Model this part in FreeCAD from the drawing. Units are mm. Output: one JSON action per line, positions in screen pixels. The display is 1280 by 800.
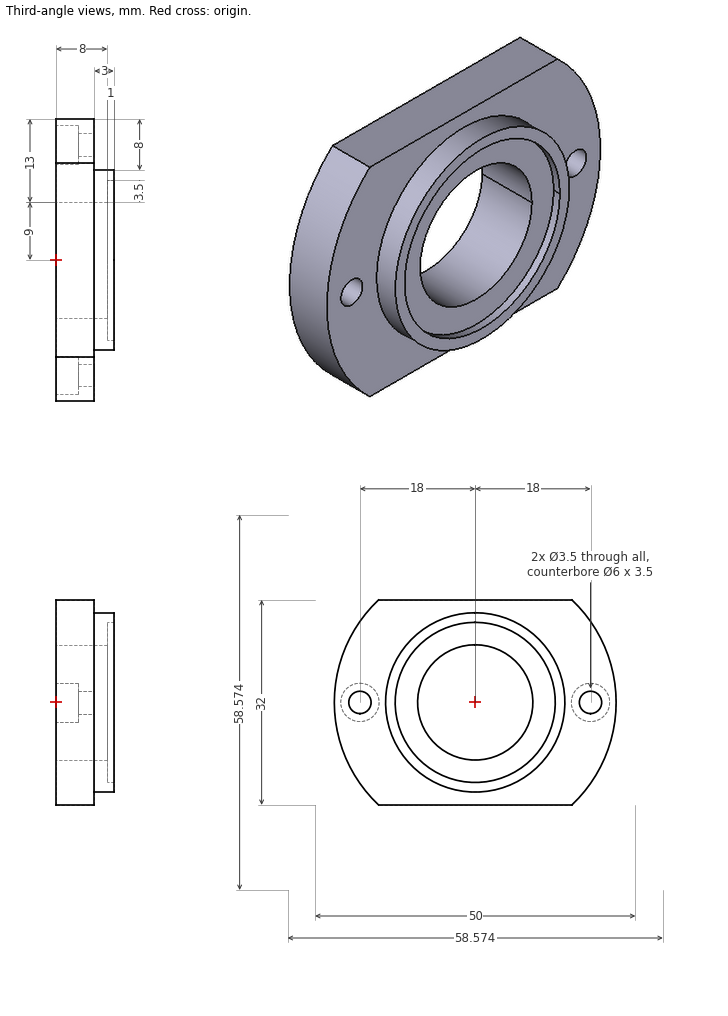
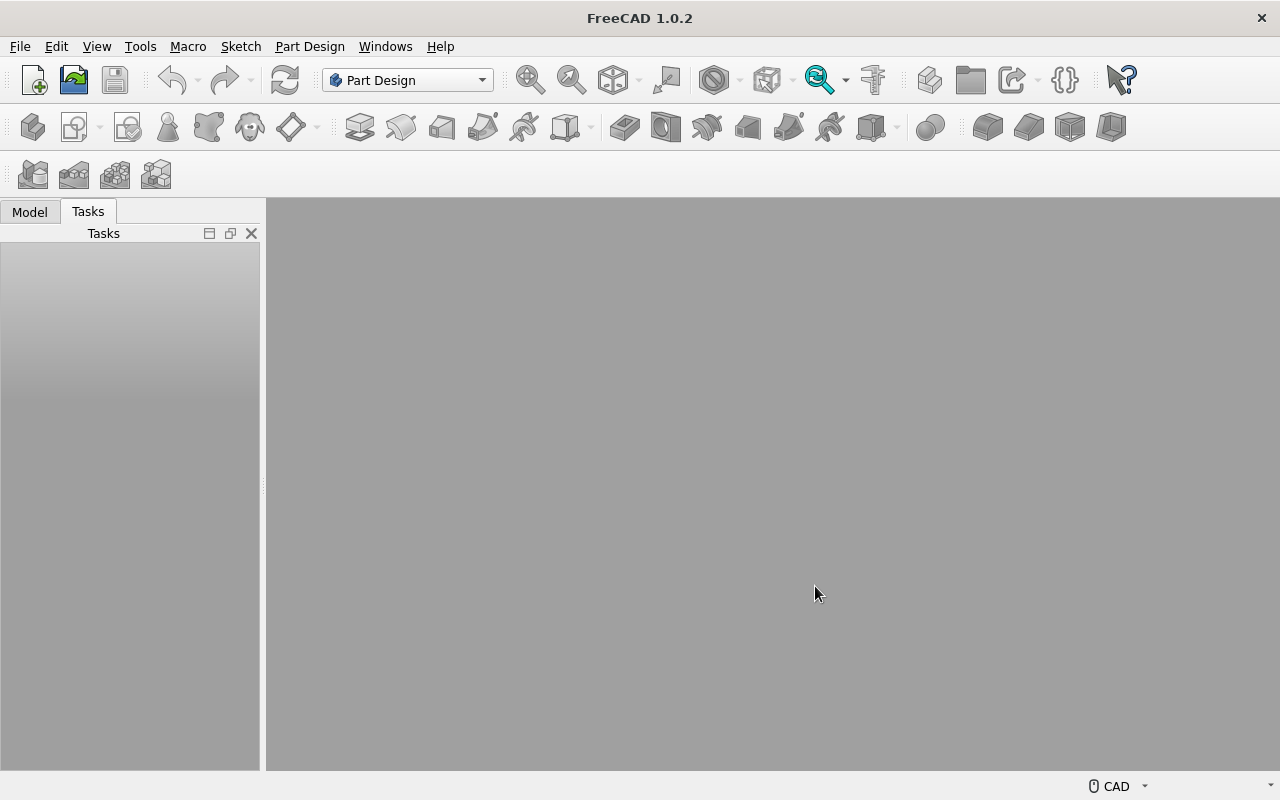
{"action": "left_click", "coordinate": [33, 80]}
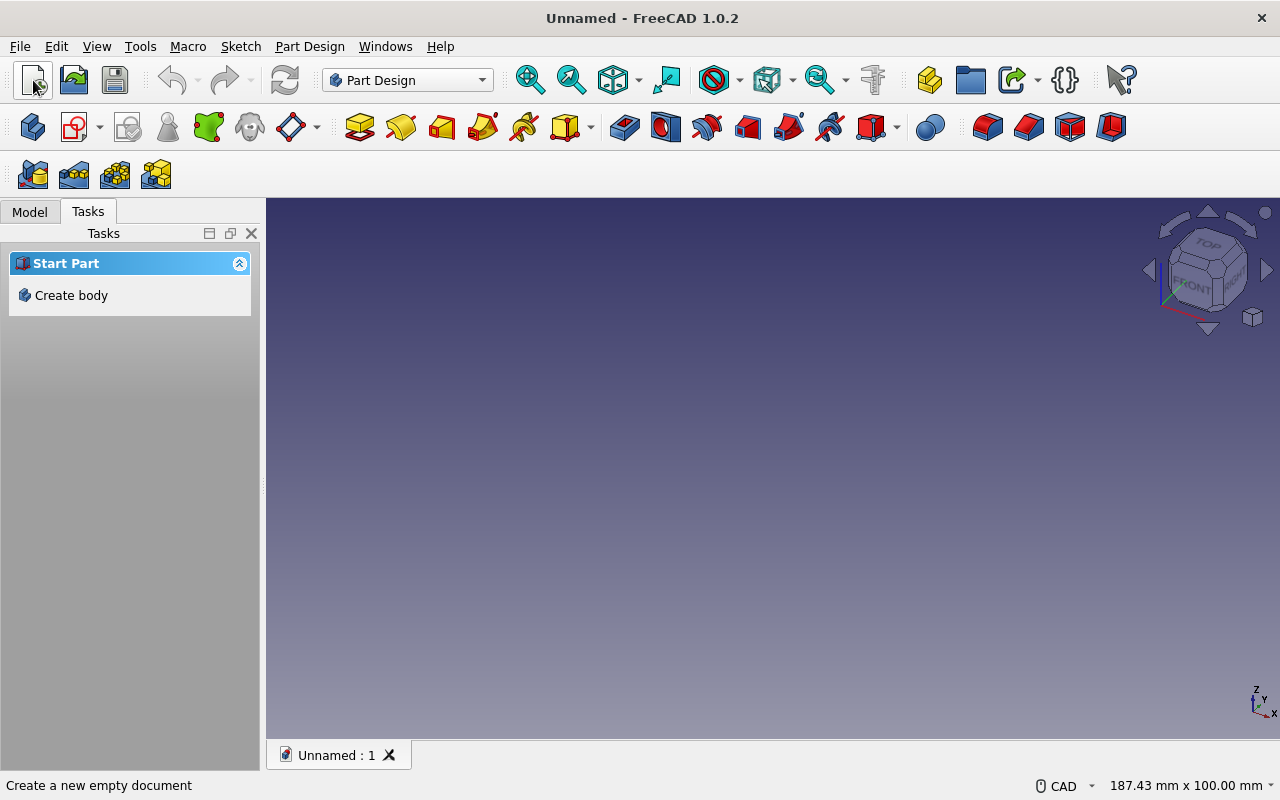
{"action": "left_click", "coordinate": [74, 128]}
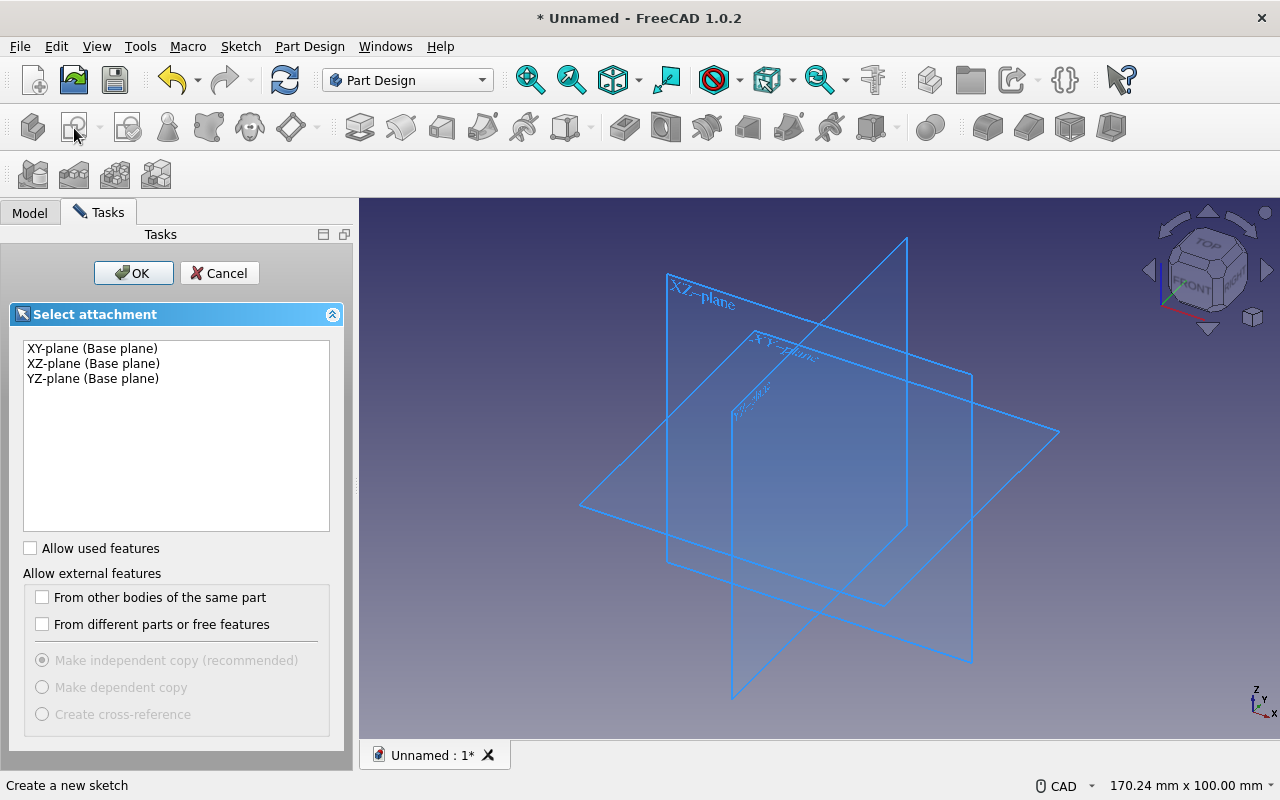
{"action": "left_click", "coordinate": [84, 348]}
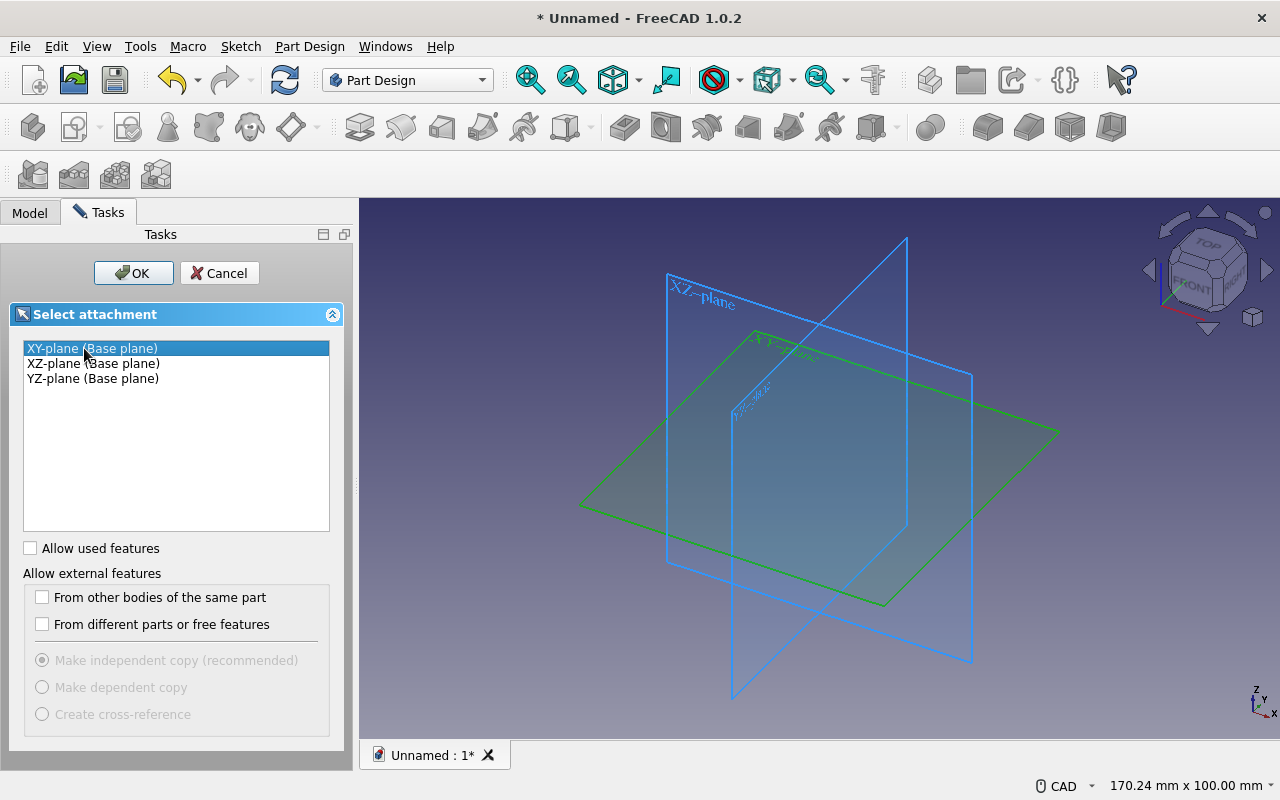
{"action": "left_click", "coordinate": [134, 273]}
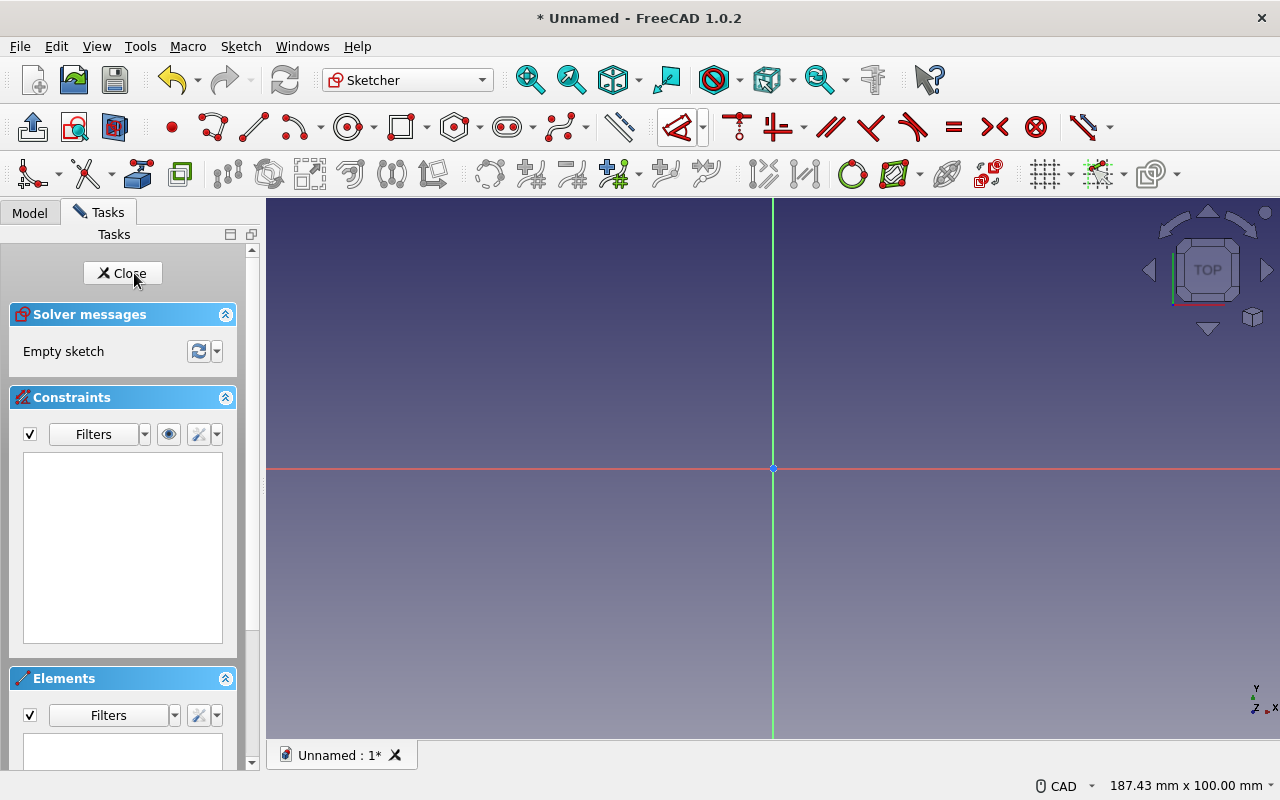
{"action": "scroll", "coordinate": [851, 374], "scroll_direction": "up", "scroll_amount": 5}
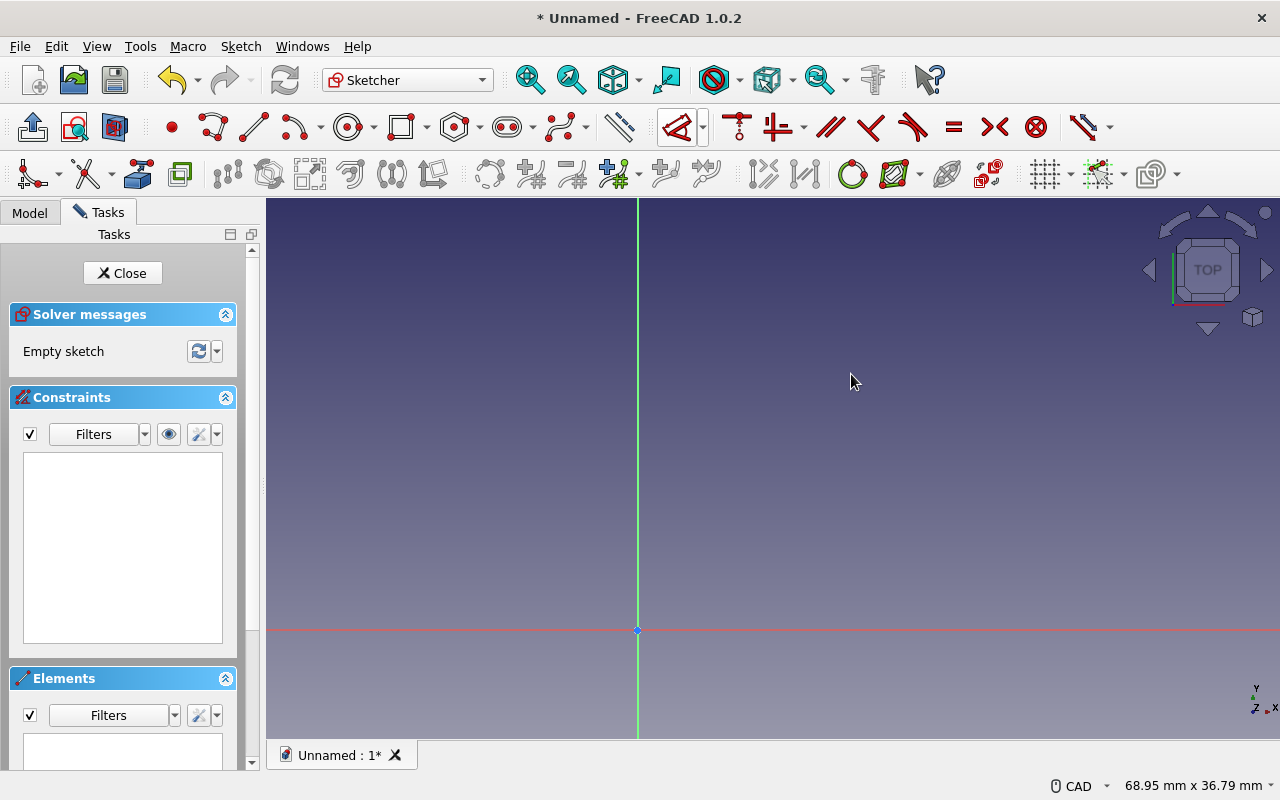
{"action": "left_click", "coordinate": [213, 128]}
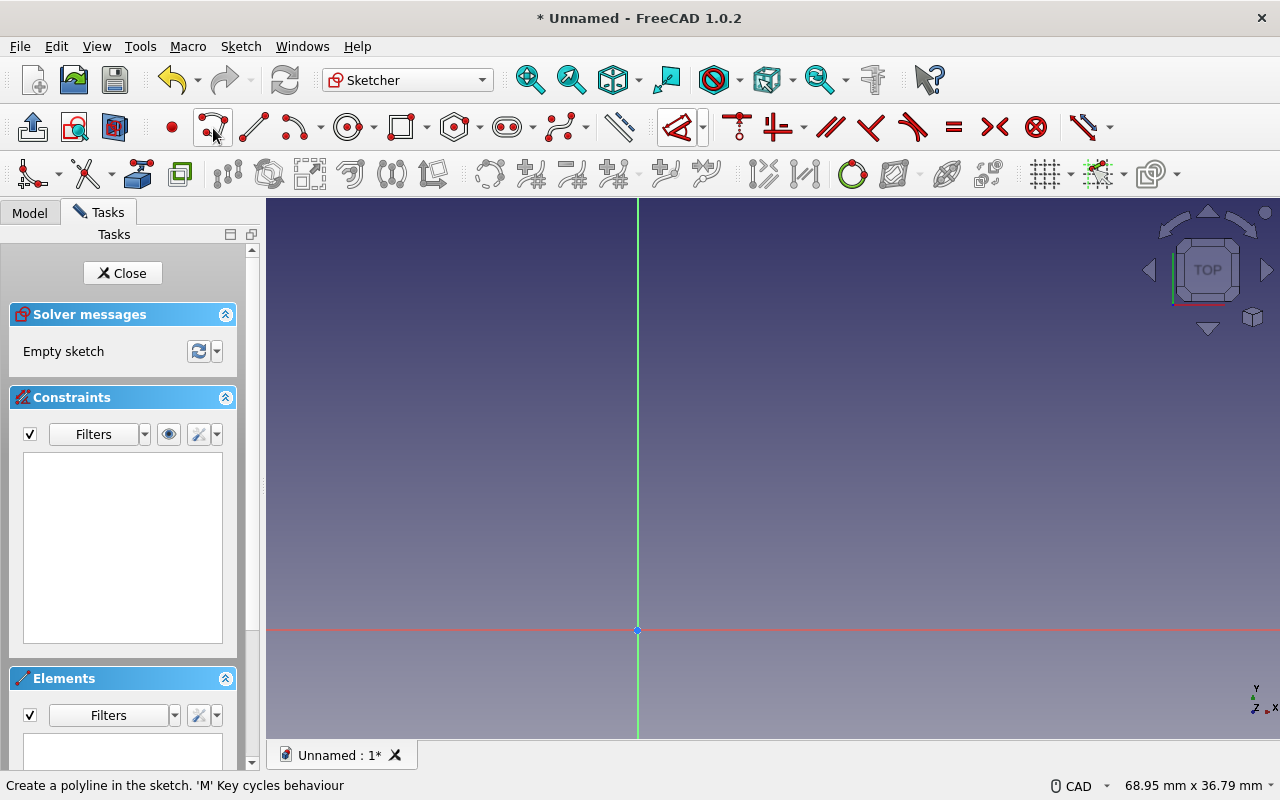
{"action": "left_click", "coordinate": [638, 498]}
{"action": "left_click", "coordinate": [756, 498]}
{"action": "left_click", "coordinate": [756, 446]}
{"action": "left_click", "coordinate": [770, 446]}
{"action": "left_click", "coordinate": [770, 424]}
{"action": "left_click", "coordinate": [726, 424]}
{"action": "left_click", "coordinate": [726, 307]}
{"action": "left_click", "coordinate": [647, 307]}
{"action": "left_click", "coordinate": [638, 499]}
{"action": "key", "text": "Escape"}
{"action": "key", "text": "Escape"}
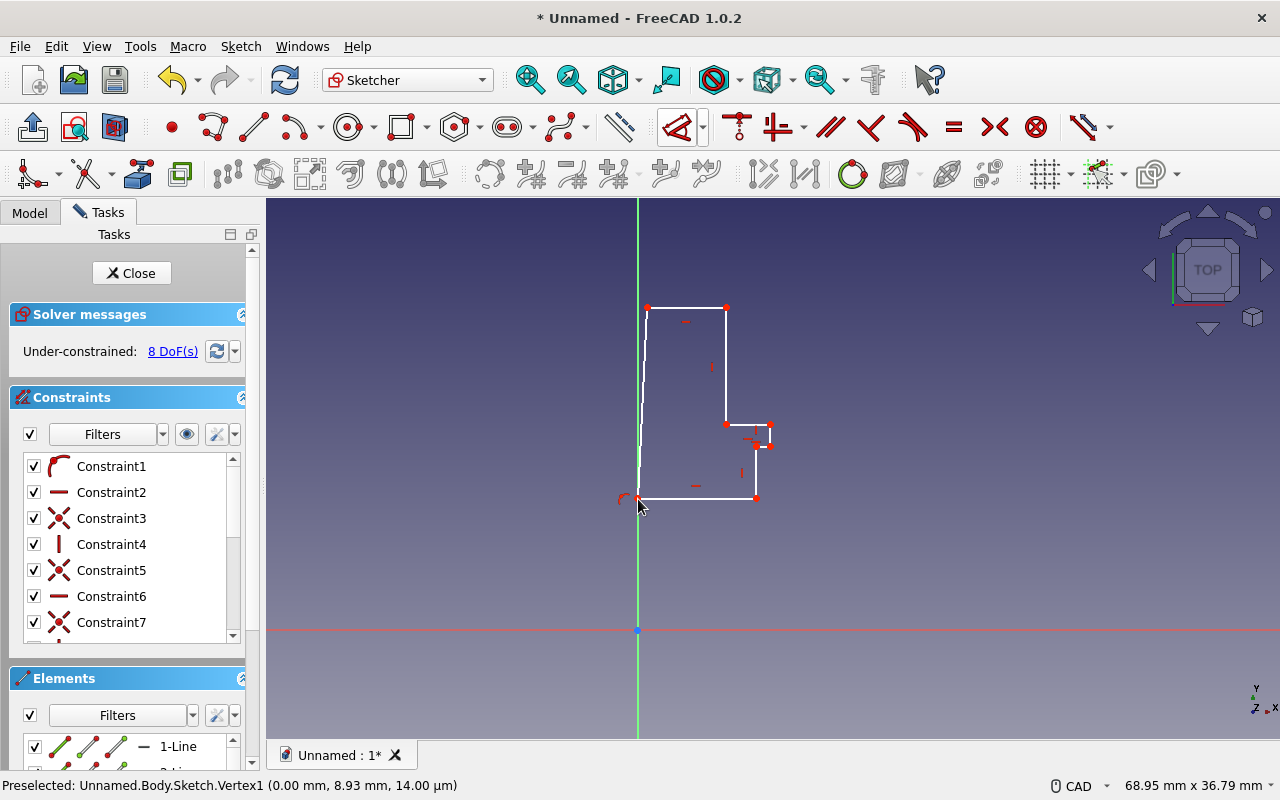
{"action": "left_click", "coordinate": [641, 442]}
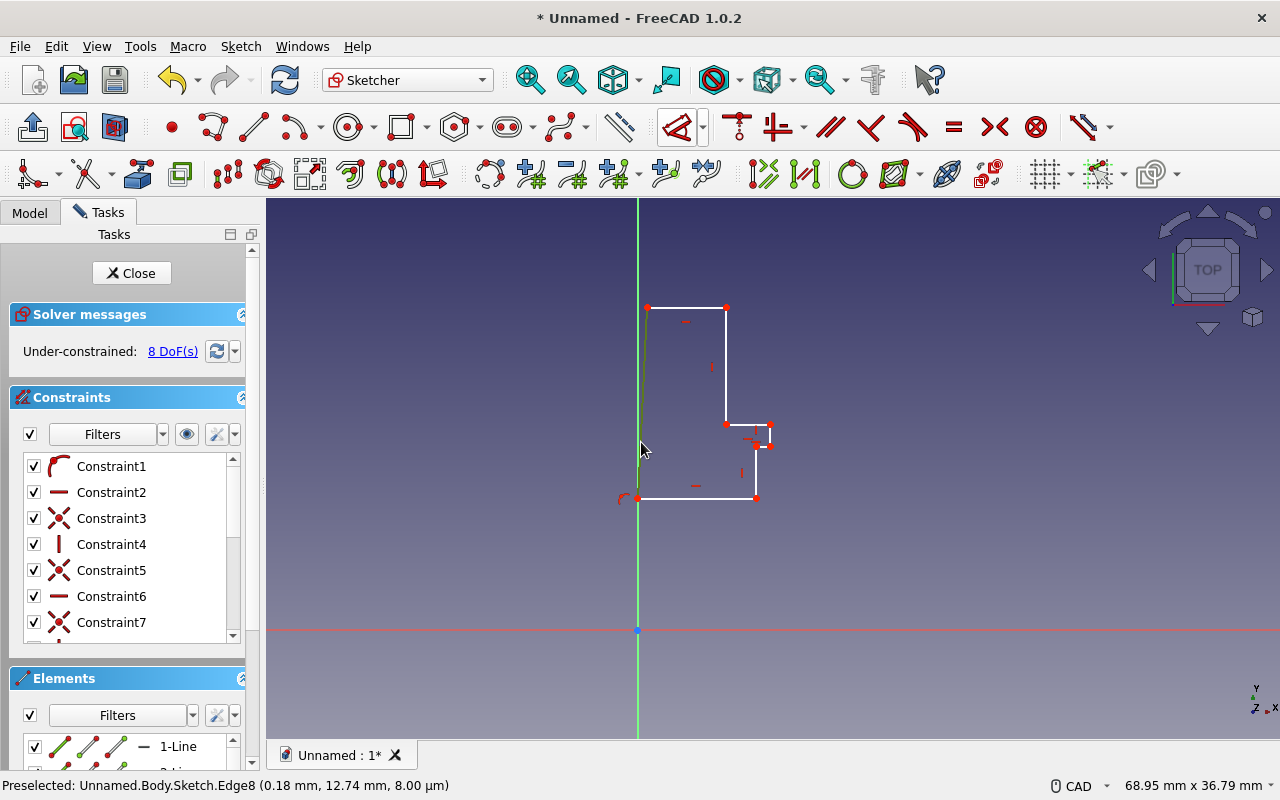
{"action": "left_click", "coordinate": [804, 128]}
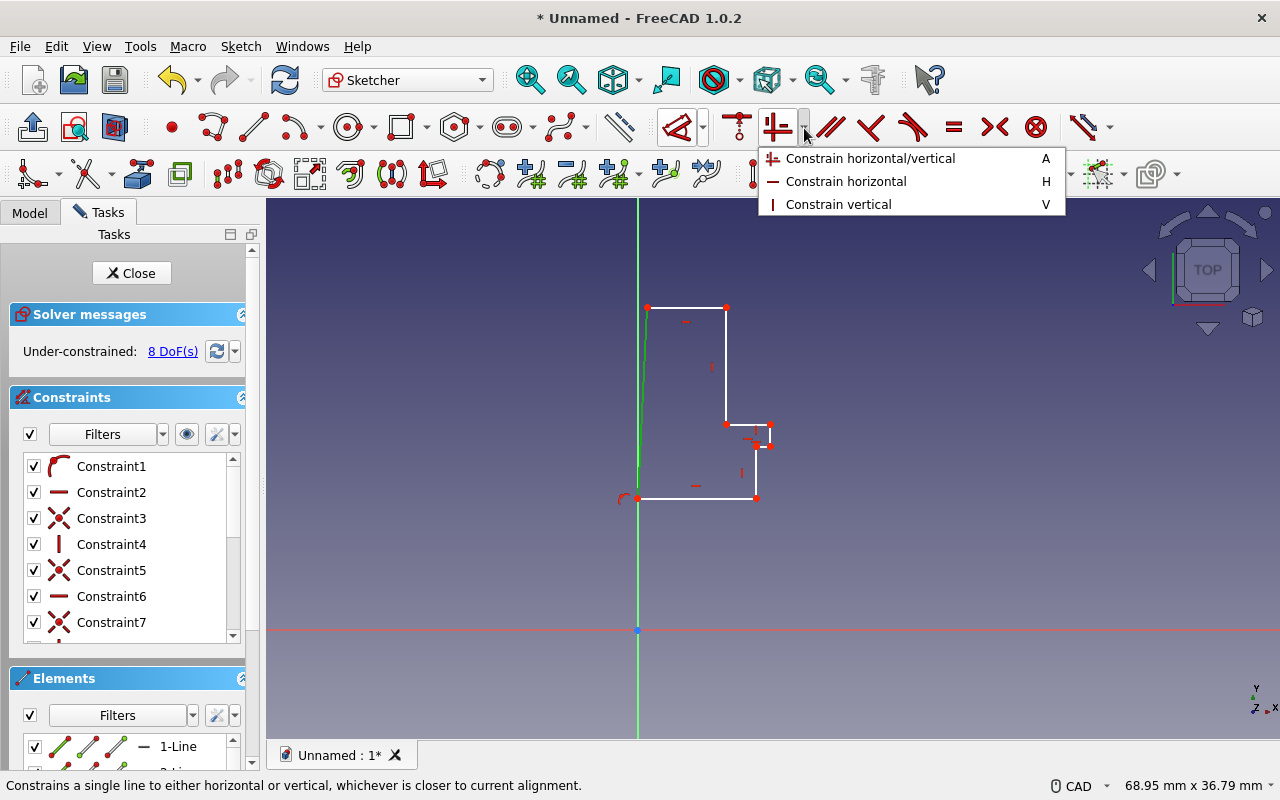
{"action": "left_click", "coordinate": [912, 204]}